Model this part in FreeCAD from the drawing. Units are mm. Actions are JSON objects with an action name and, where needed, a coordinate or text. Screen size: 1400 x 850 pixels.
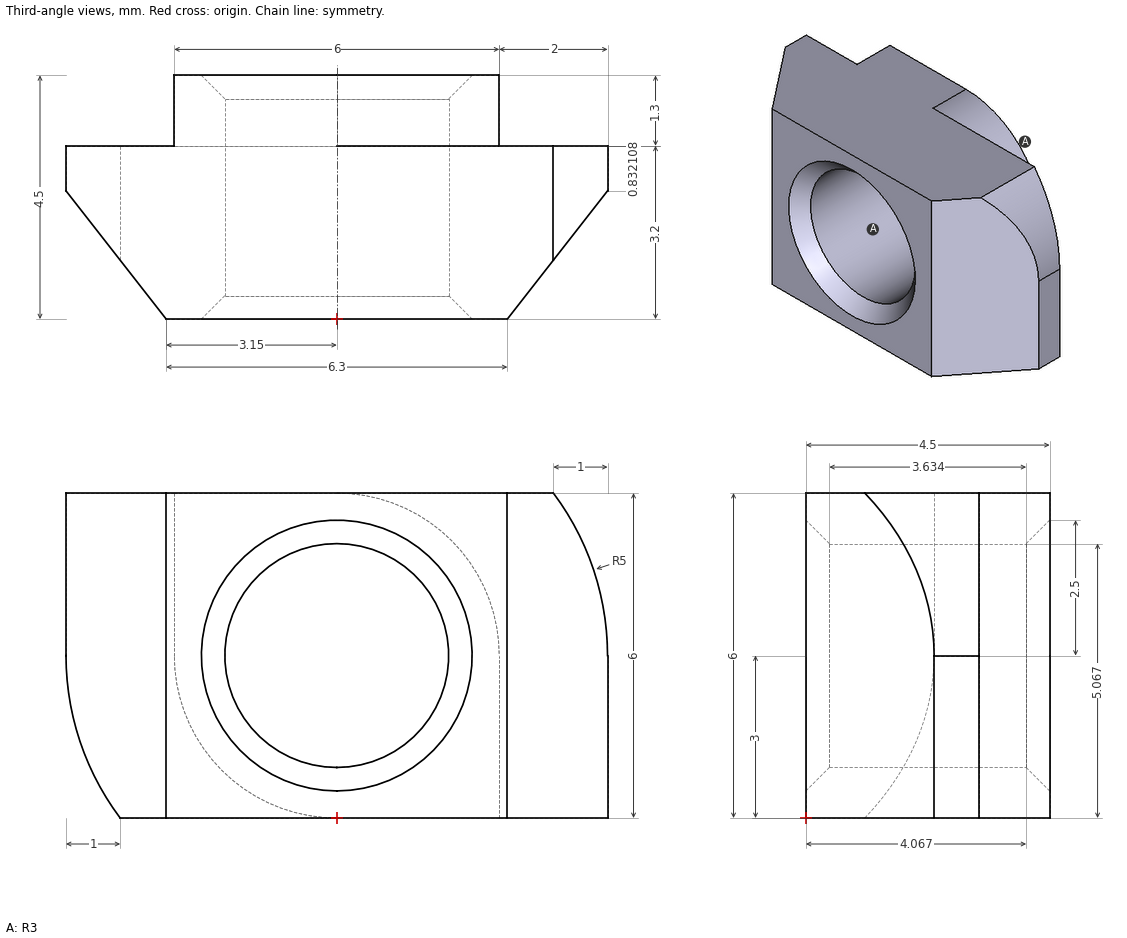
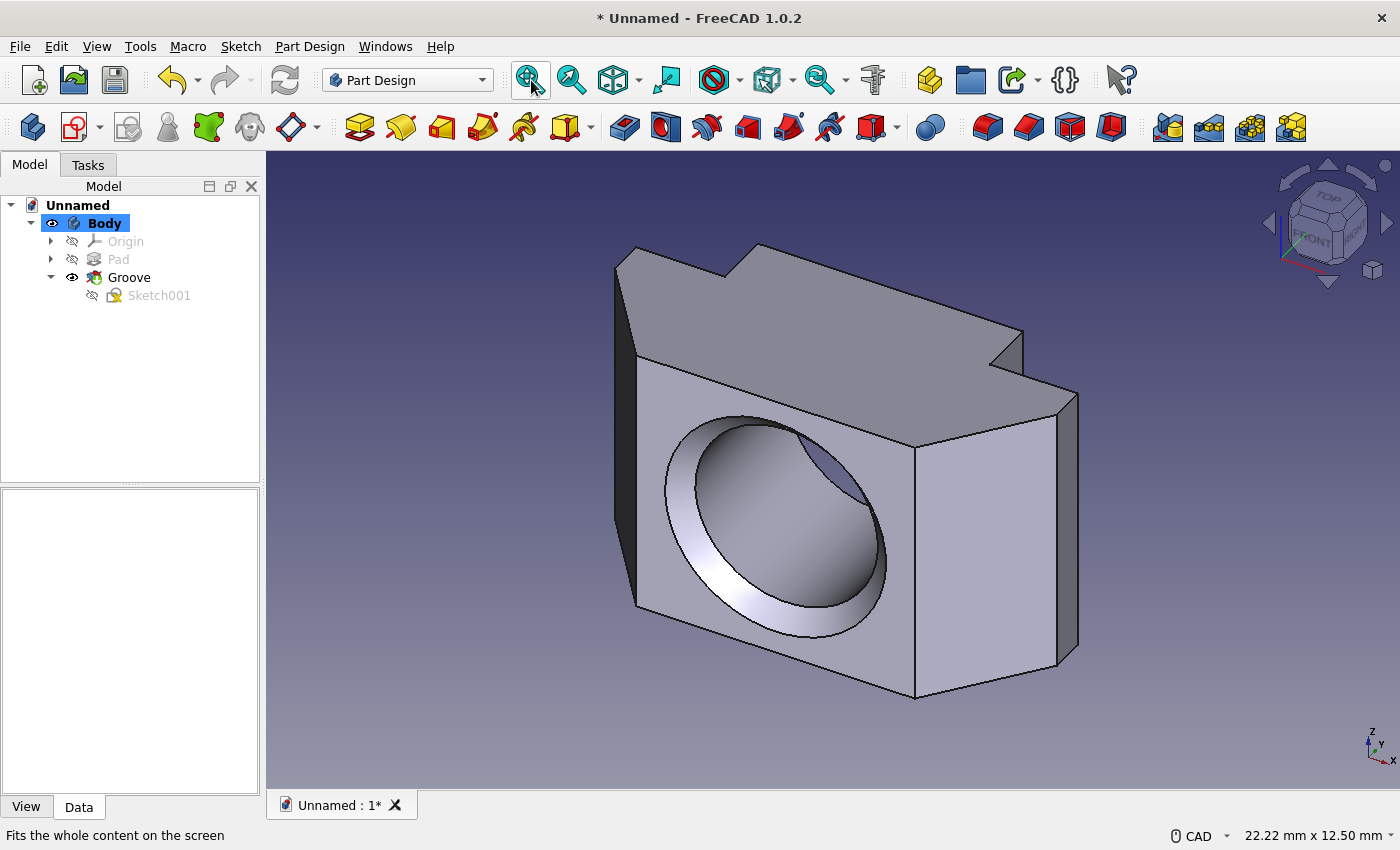
{"action": "key", "text": "4"}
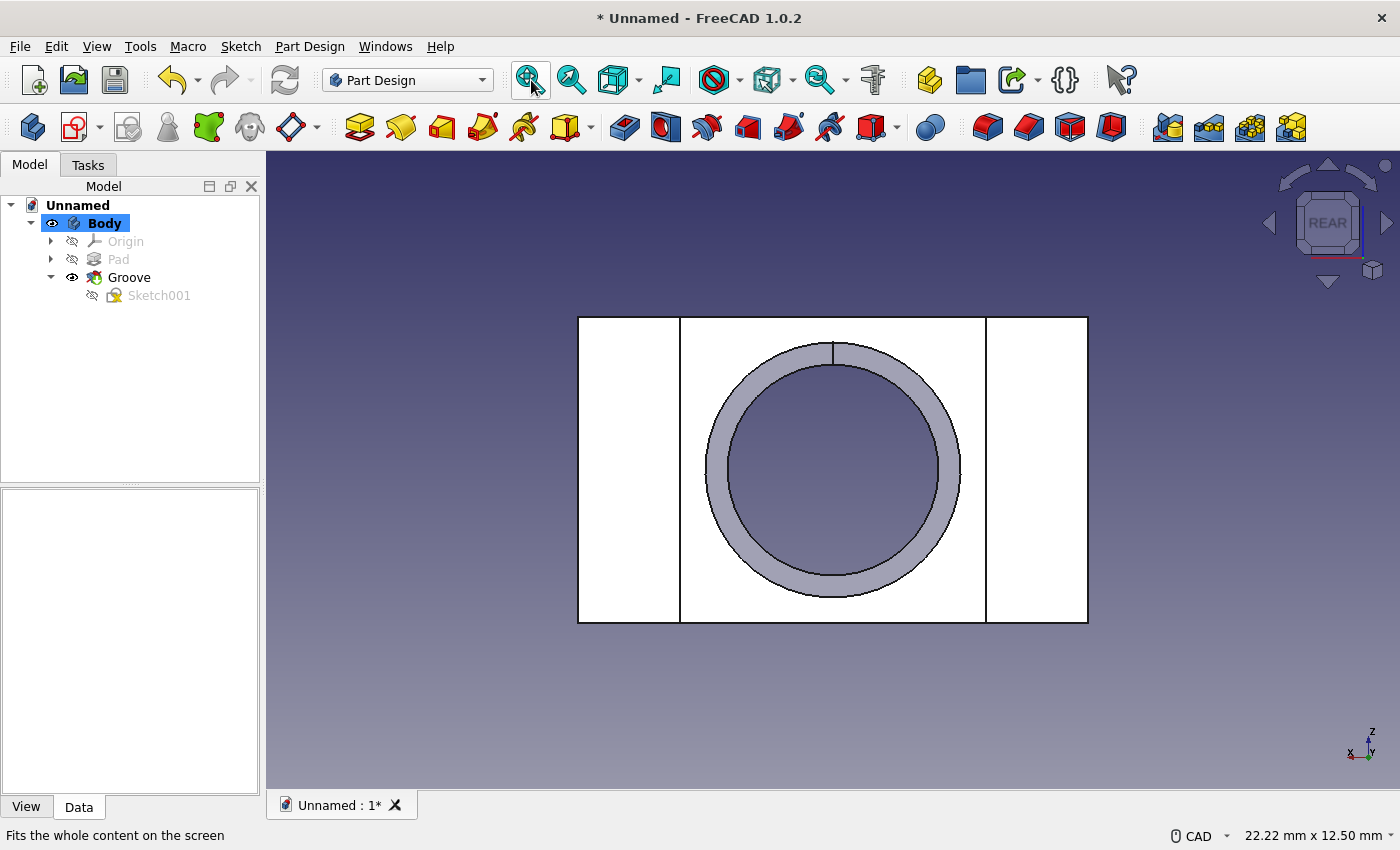
{"action": "left_click", "coordinate": [746, 338]}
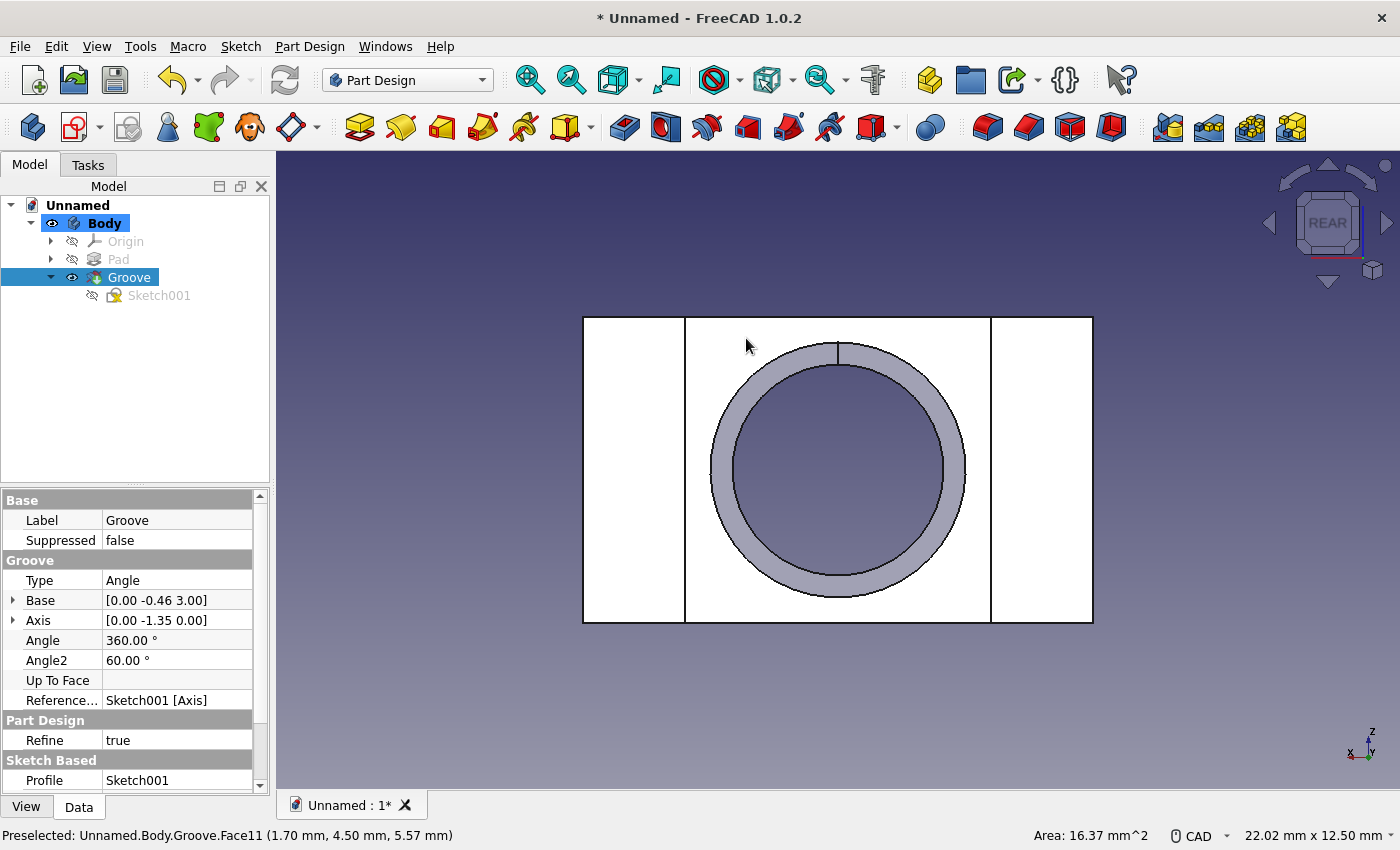
{"action": "left_click", "coordinate": [74, 128]}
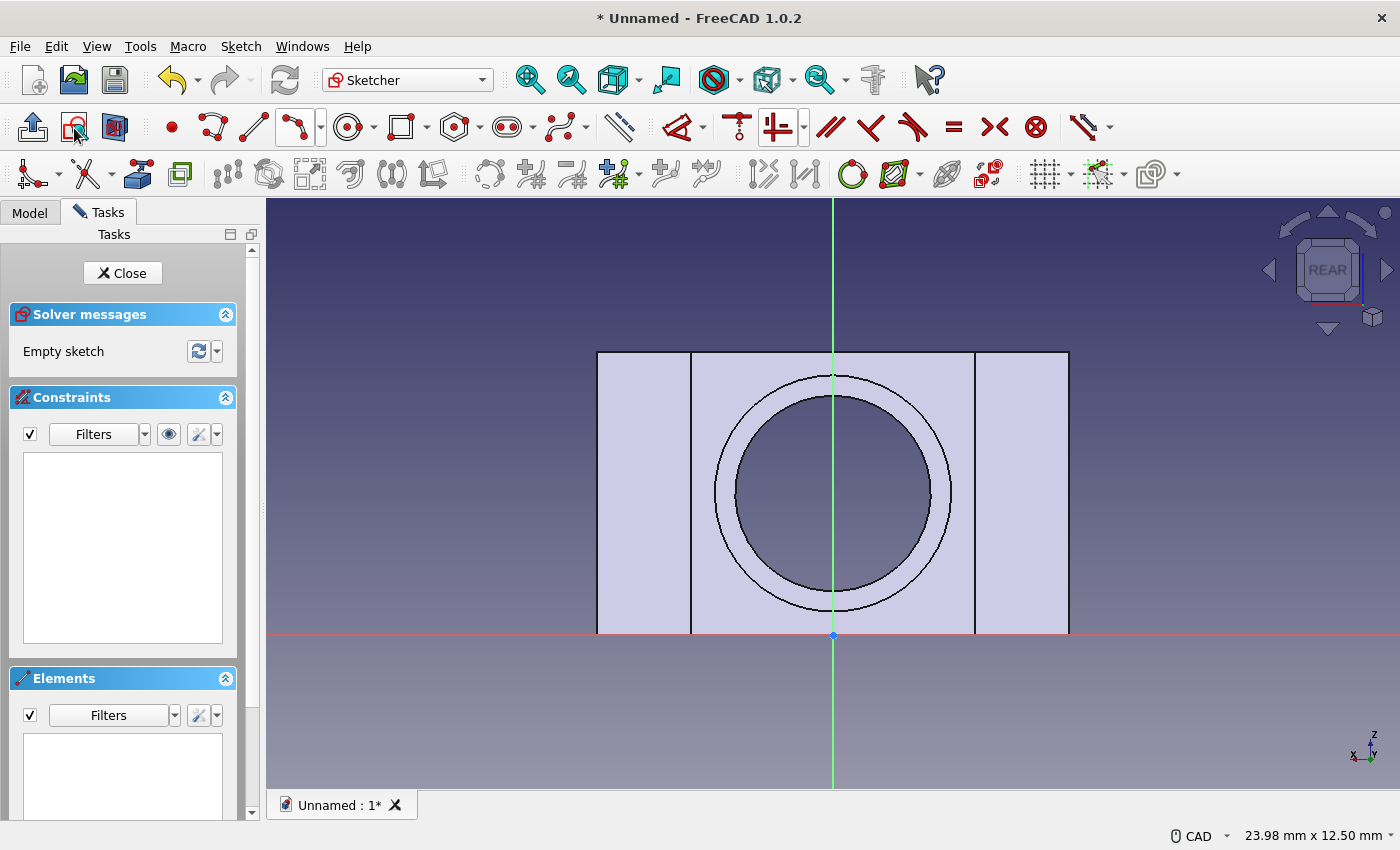
{"action": "left_click", "coordinate": [213, 128]}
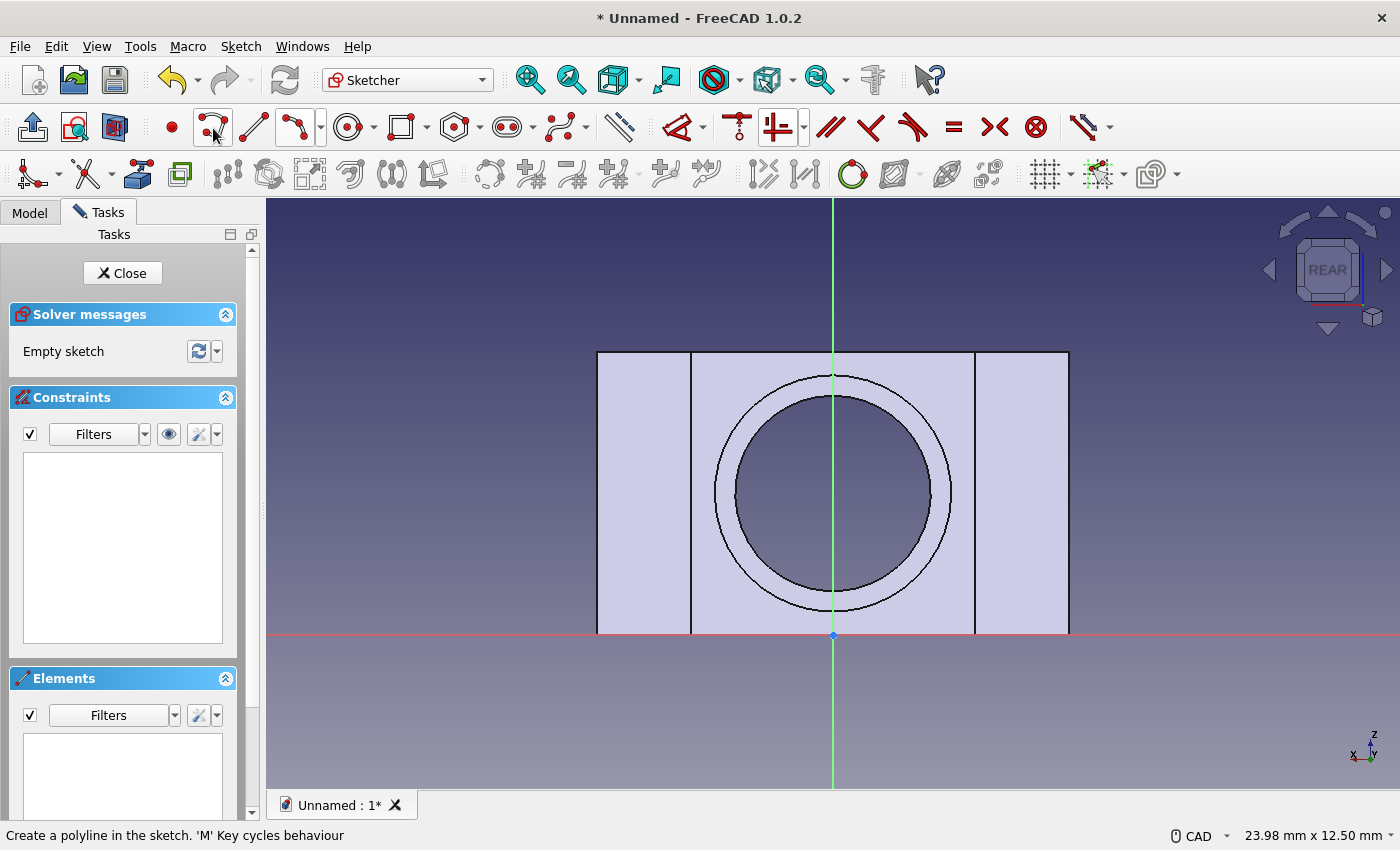
{"action": "left_click", "coordinate": [644, 352]}
{"action": "left_click", "coordinate": [597, 352]}
{"action": "left_click", "coordinate": [597, 493]}
{"action": "right_click", "coordinate": [597, 493]}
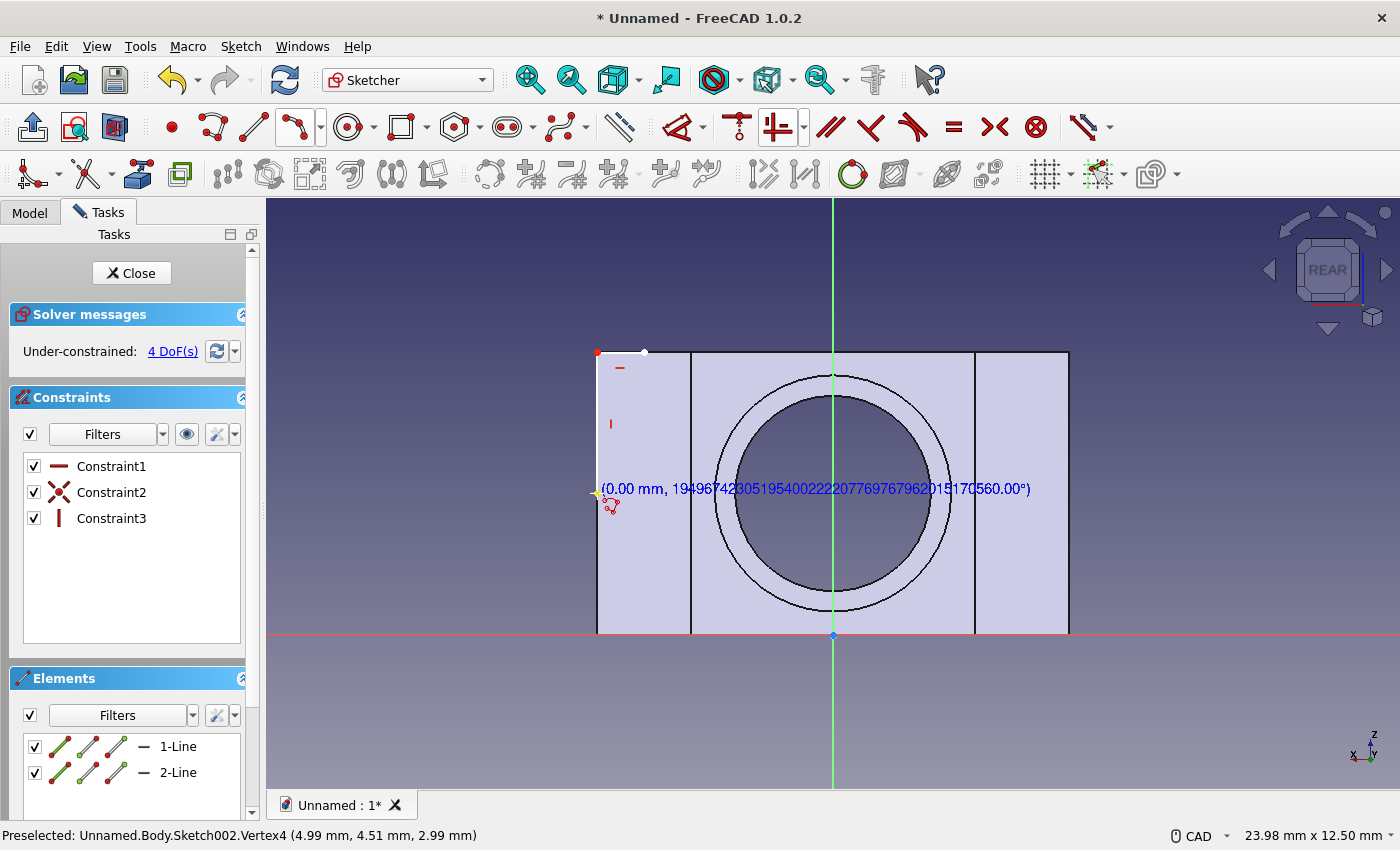
{"action": "left_click", "coordinate": [294, 128]}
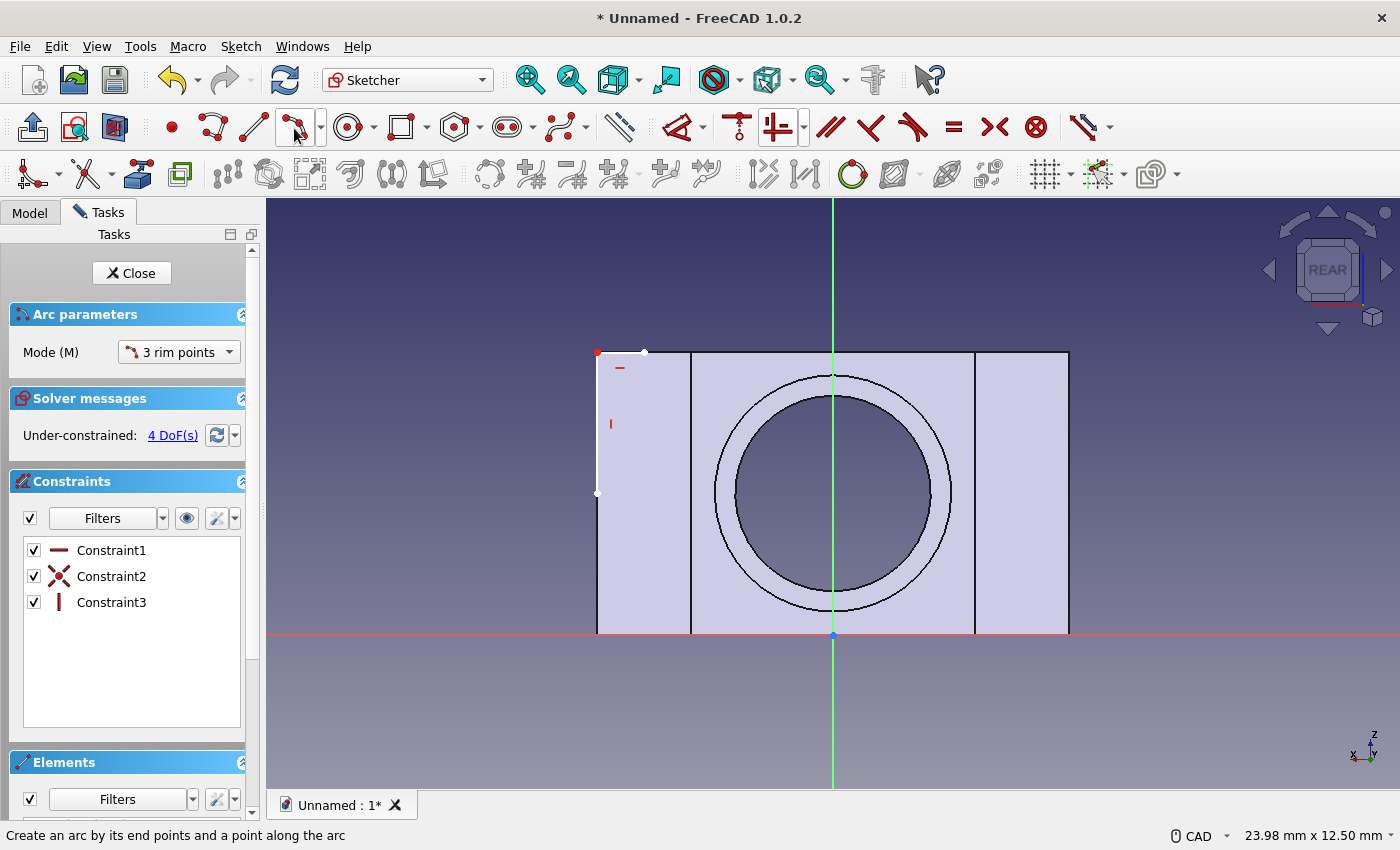
{"action": "left_click", "coordinate": [597, 494]}
{"action": "left_click", "coordinate": [644, 353]}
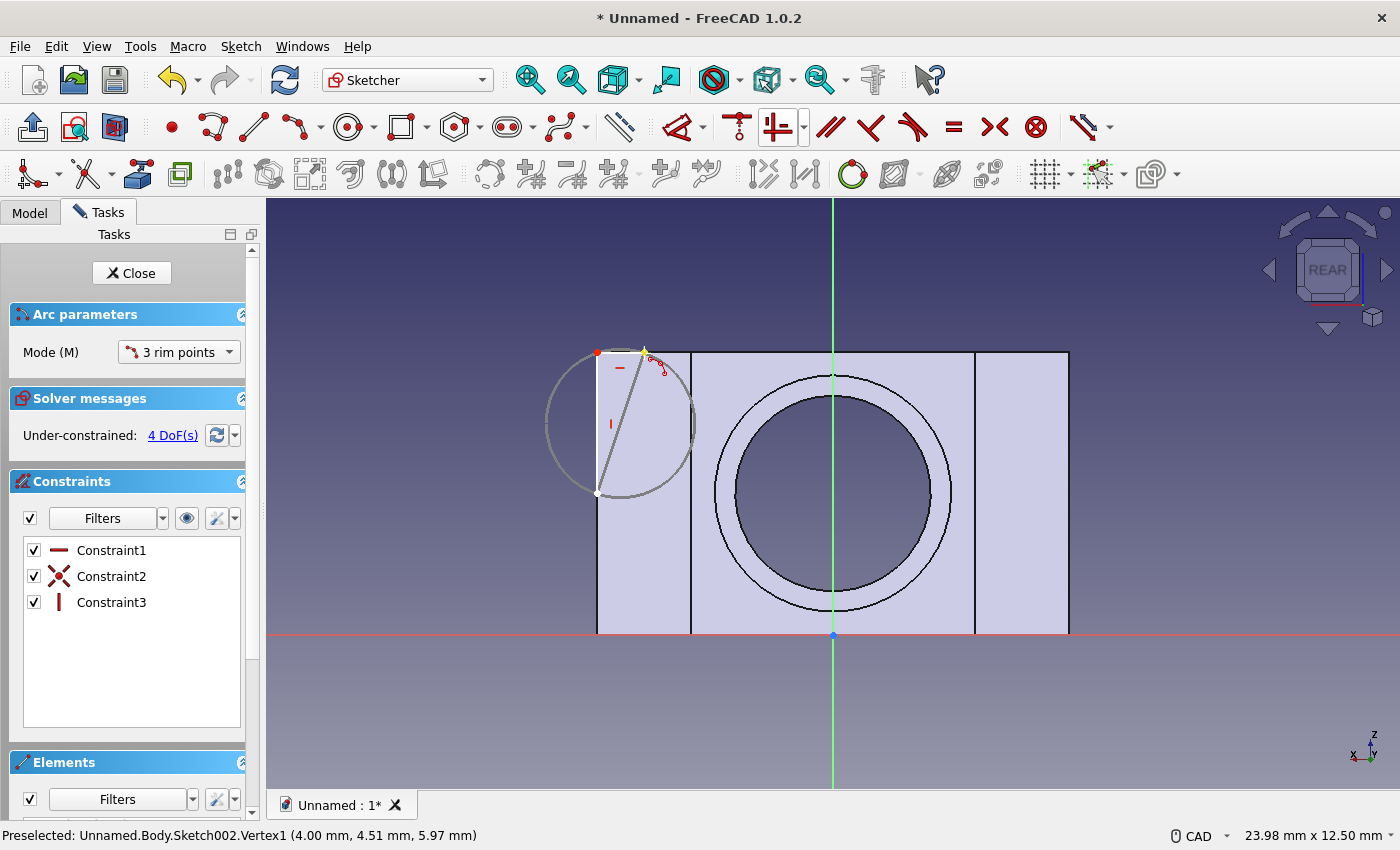
{"action": "scroll", "coordinate": [609, 419], "scroll_direction": "up", "scroll_amount": 2}